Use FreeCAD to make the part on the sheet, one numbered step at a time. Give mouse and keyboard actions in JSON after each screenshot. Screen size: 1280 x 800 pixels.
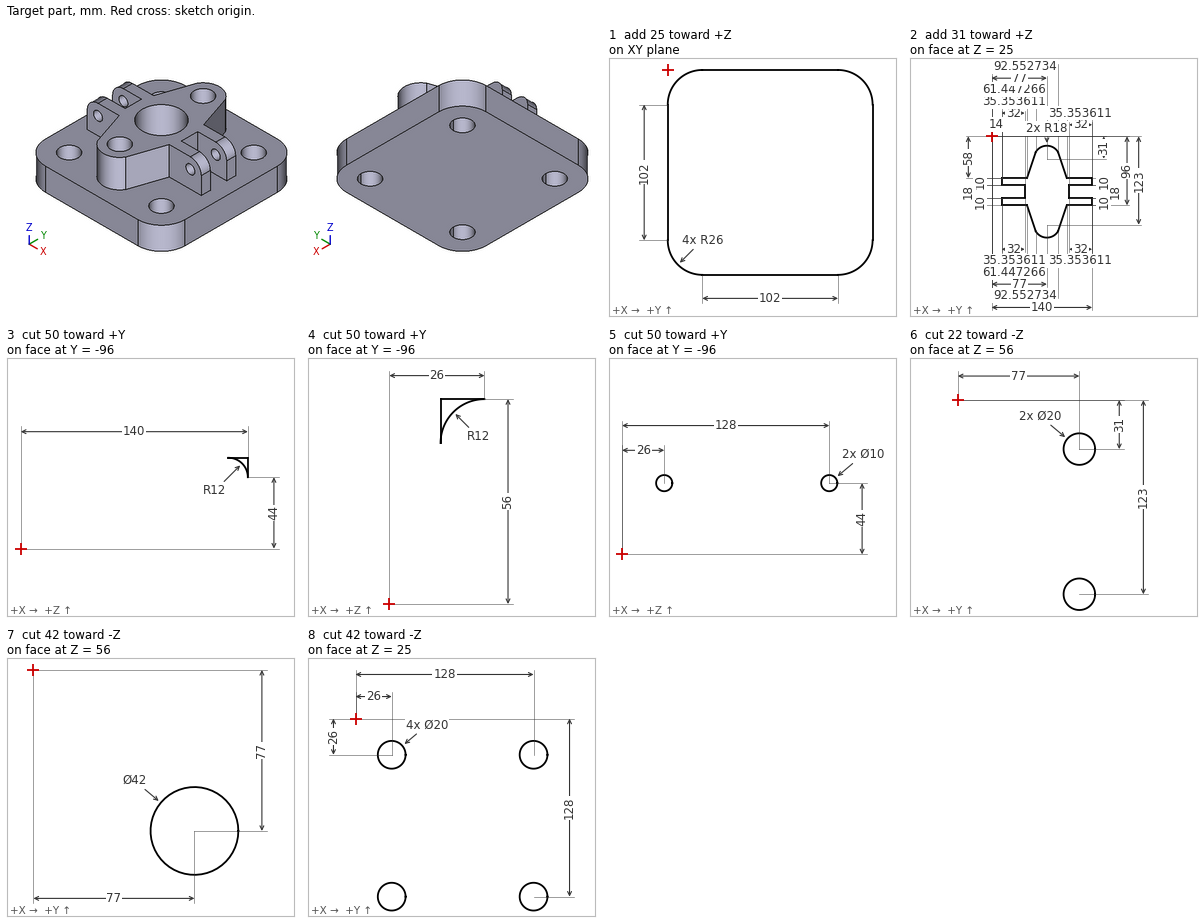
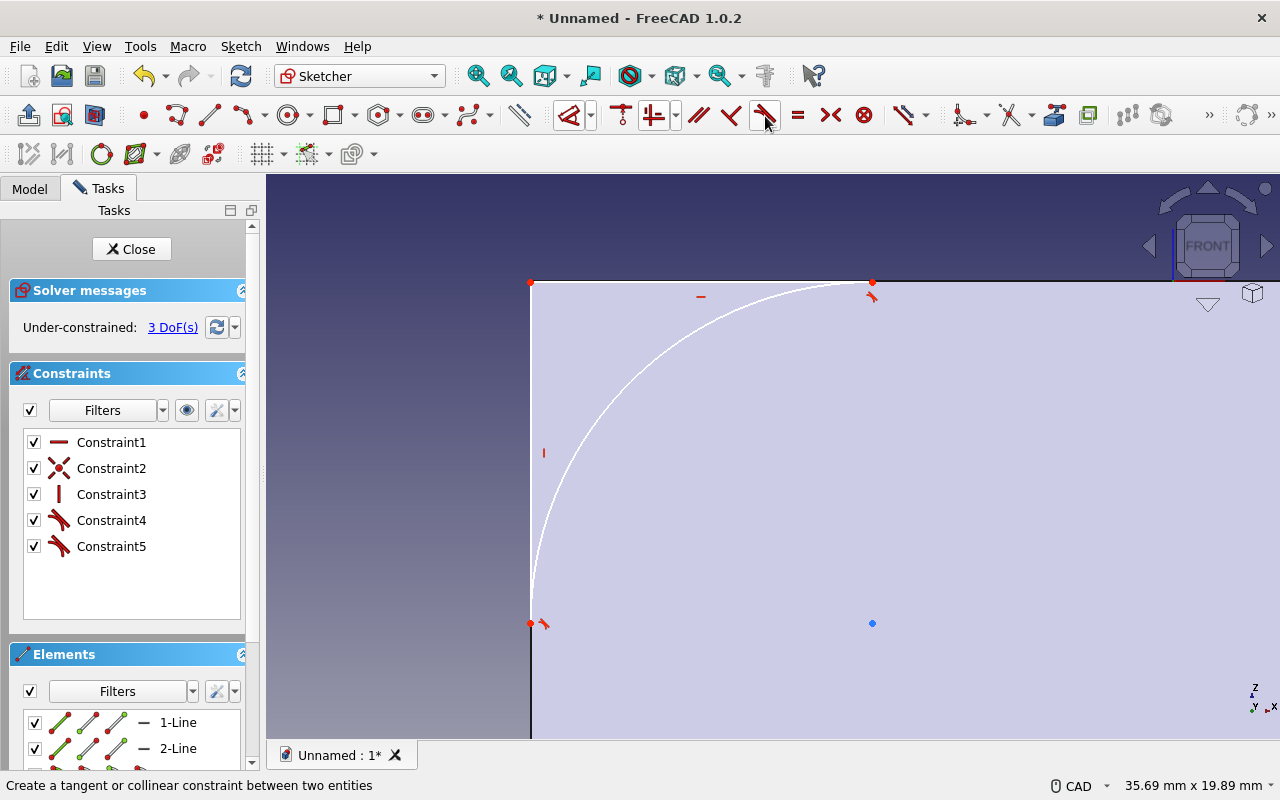
{"action": "left_click", "coordinate": [717, 319]}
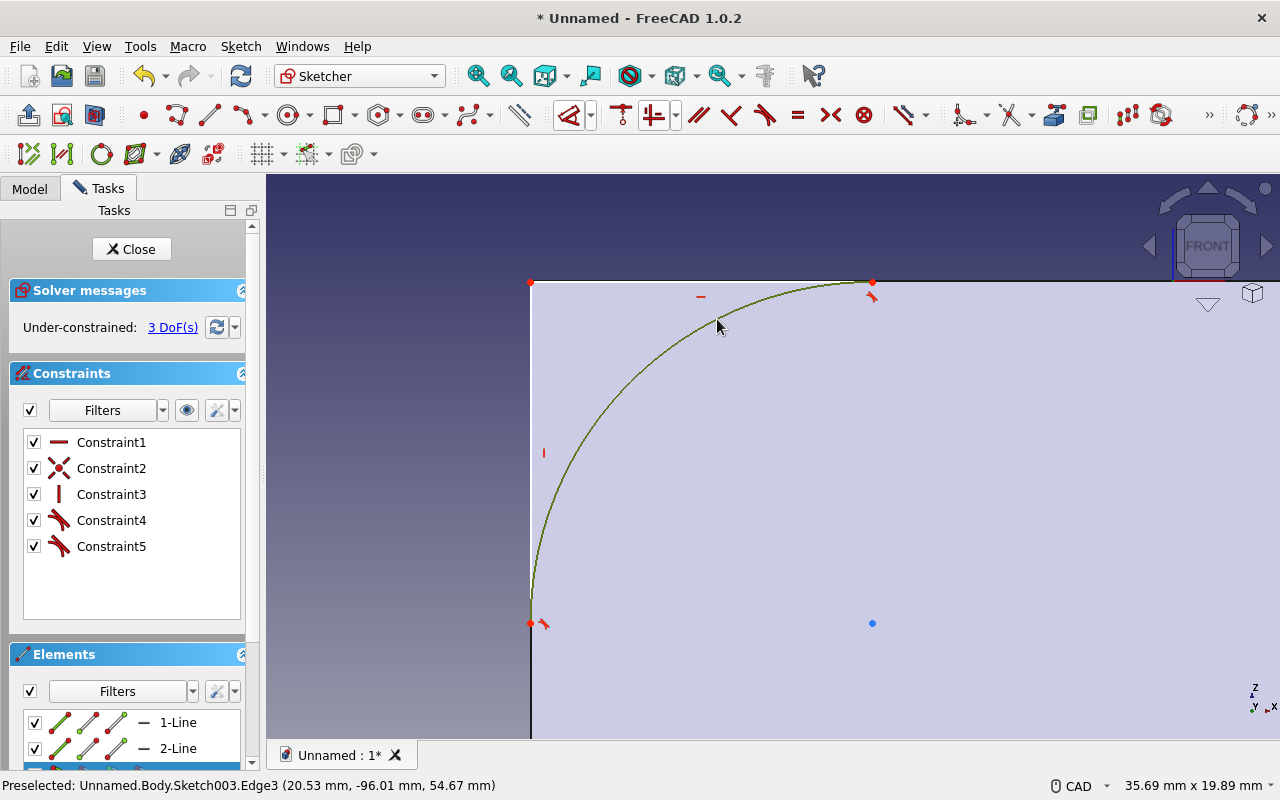
{"action": "key", "text": "k r"}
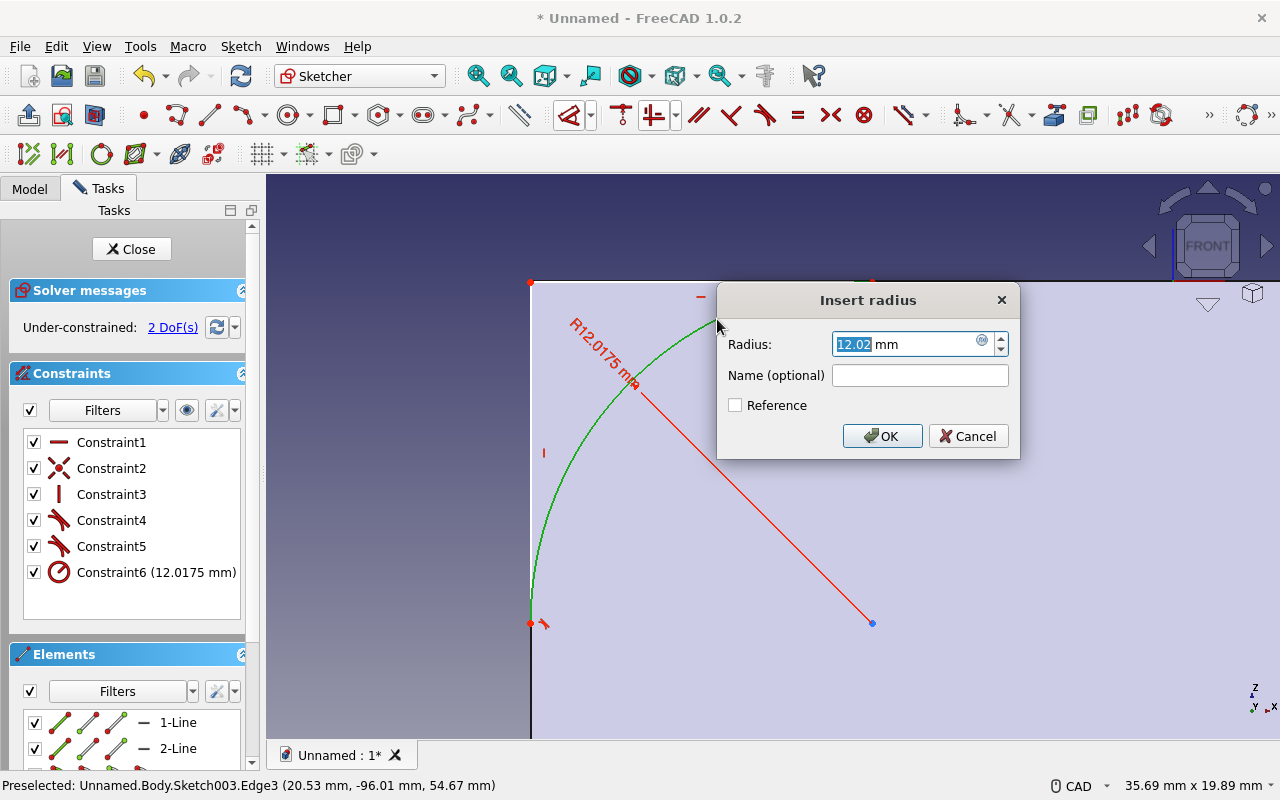
{"action": "type", "text": "12"}
{"action": "key", "text": "Return"}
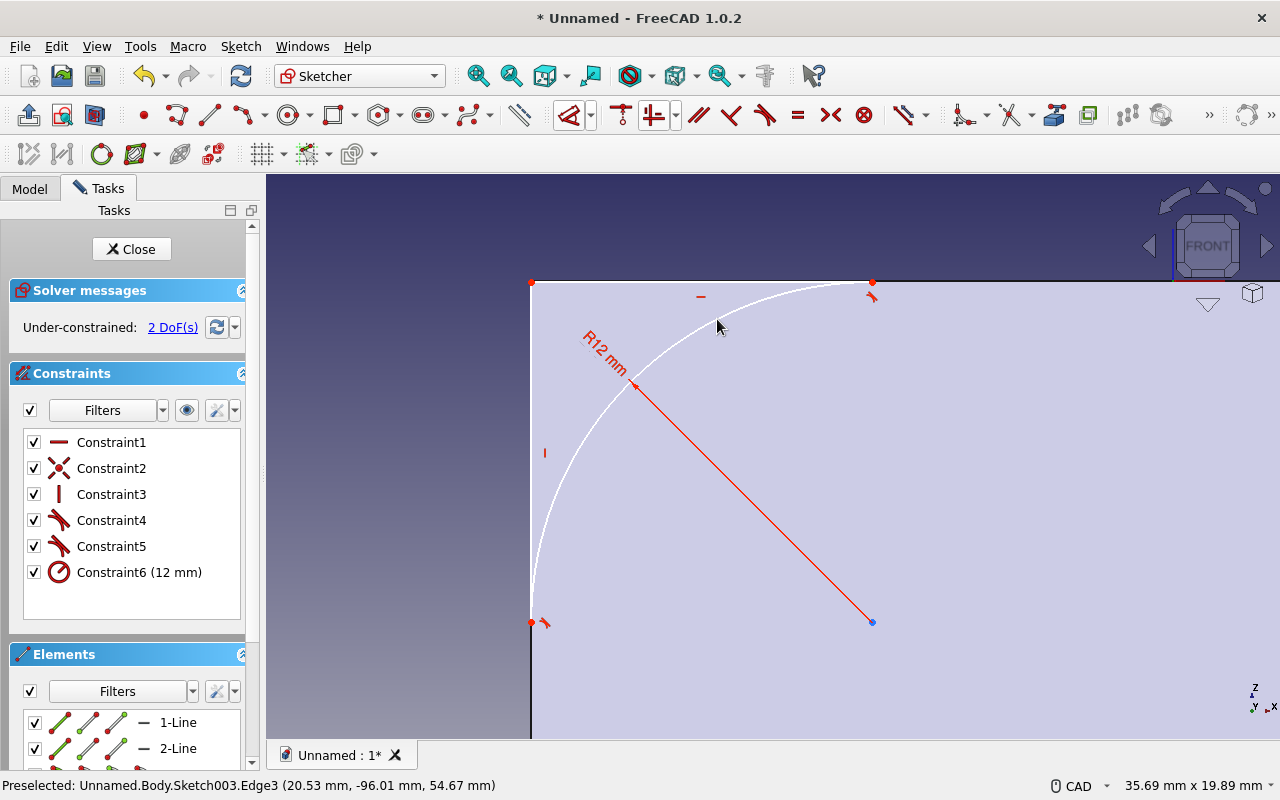
{"action": "left_click", "coordinate": [872, 282]}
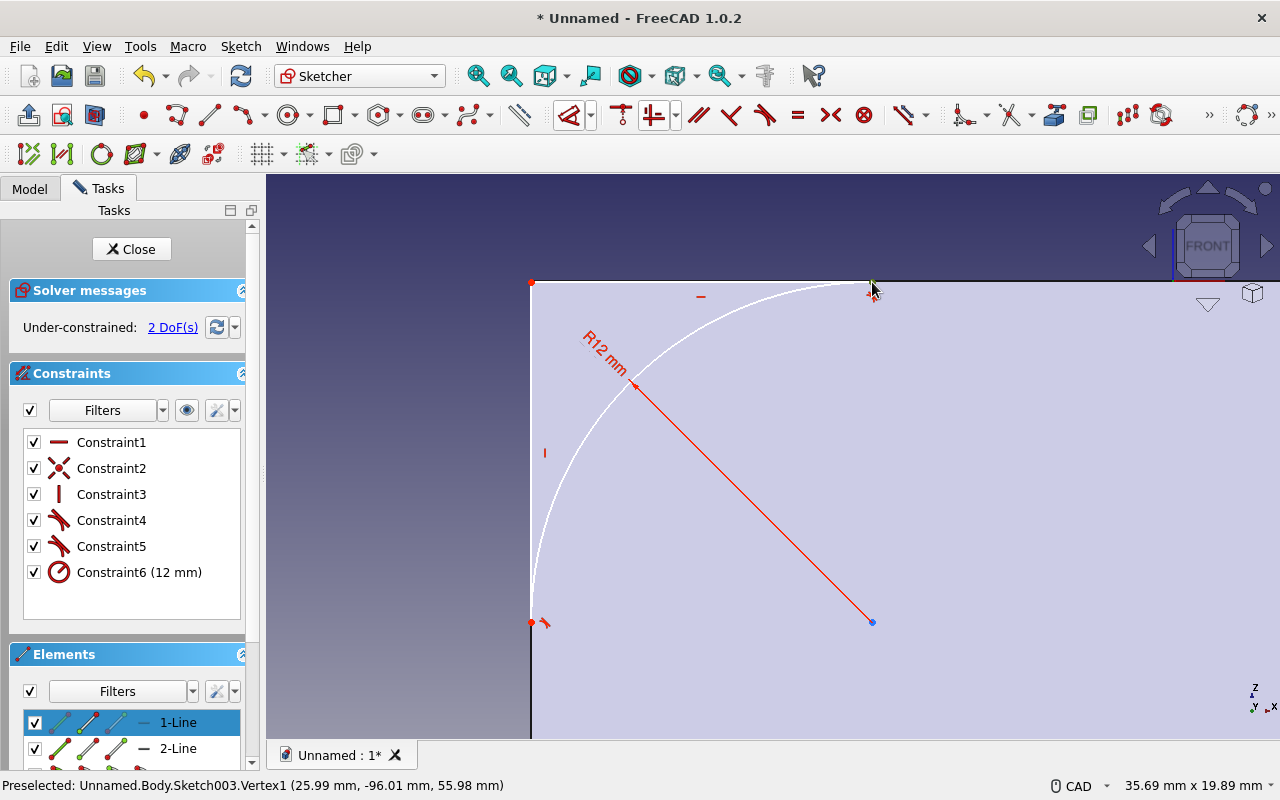
{"action": "key", "text": "l"}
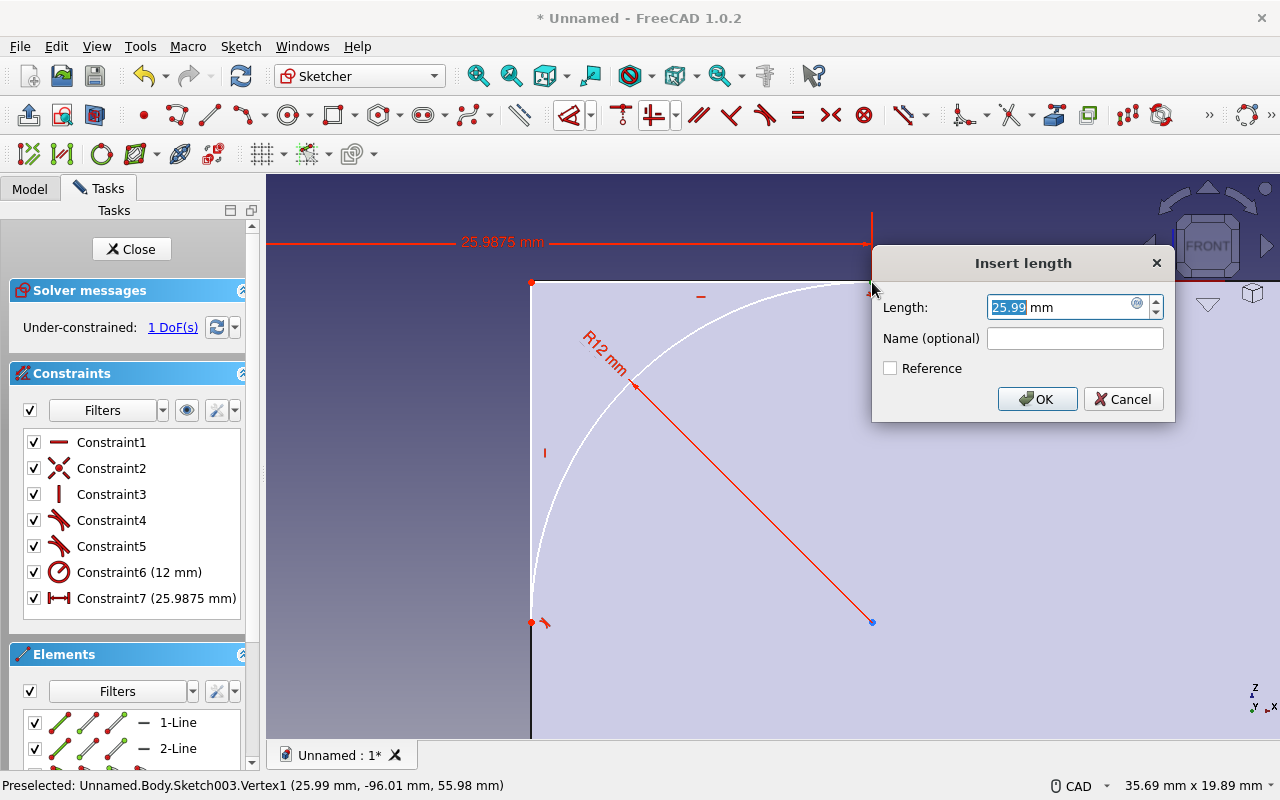
{"action": "type", "text": "26"}
{"action": "key", "text": "Return"}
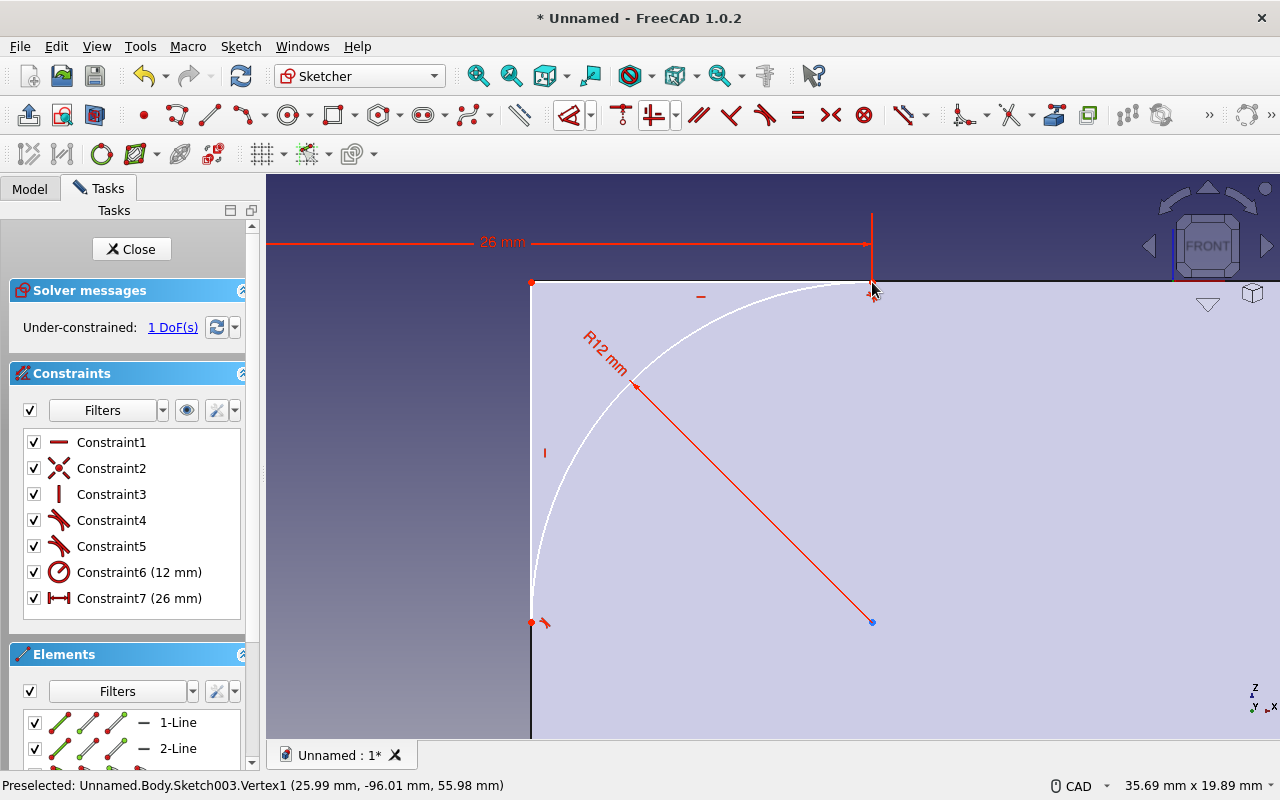
{"action": "left_click", "coordinate": [872, 282]}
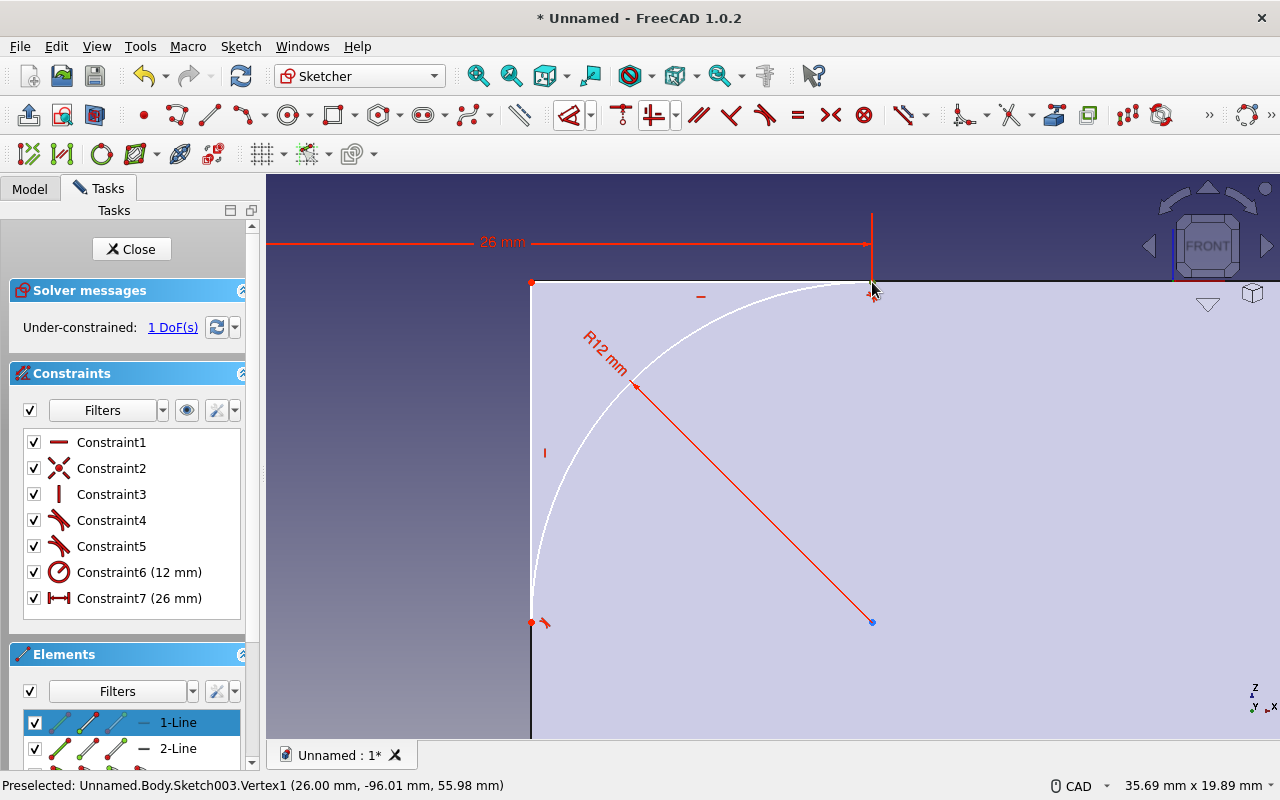
{"action": "left_click", "coordinate": [590, 116]}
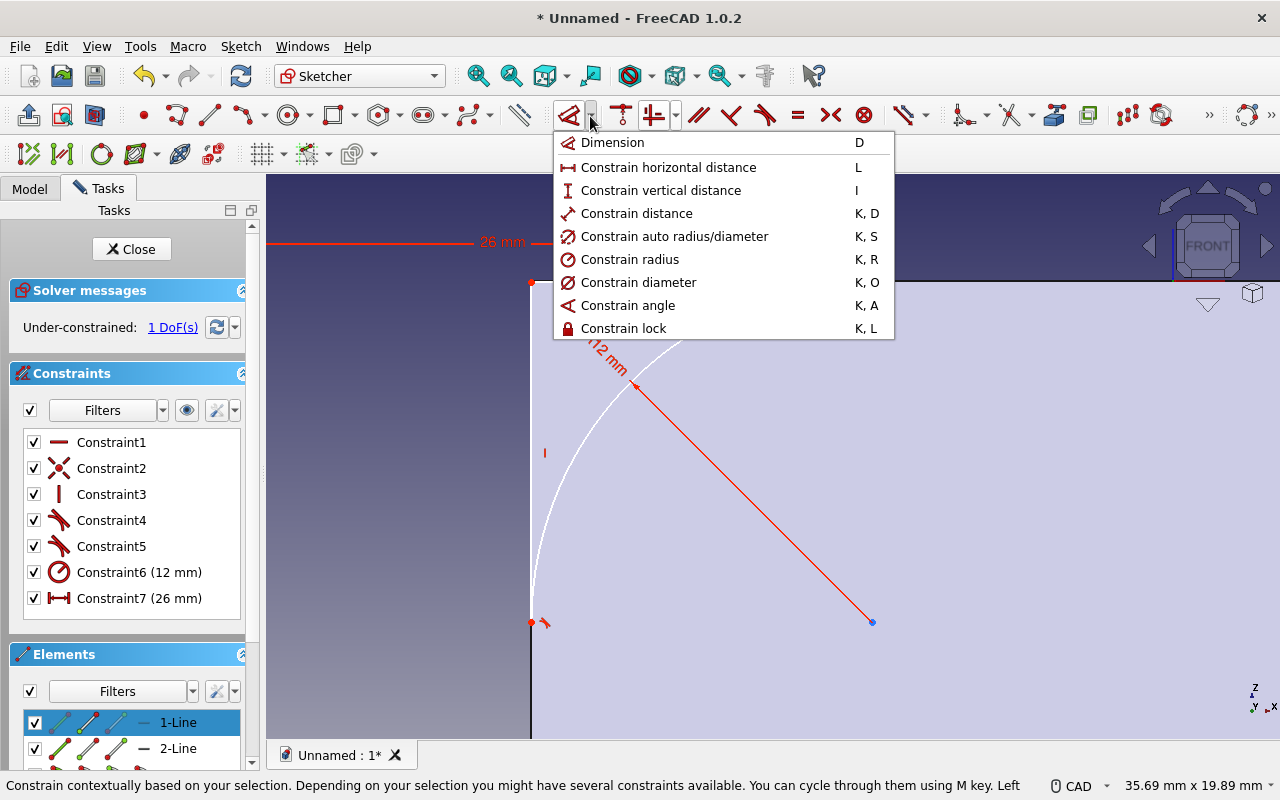
{"action": "left_click", "coordinate": [724, 190]}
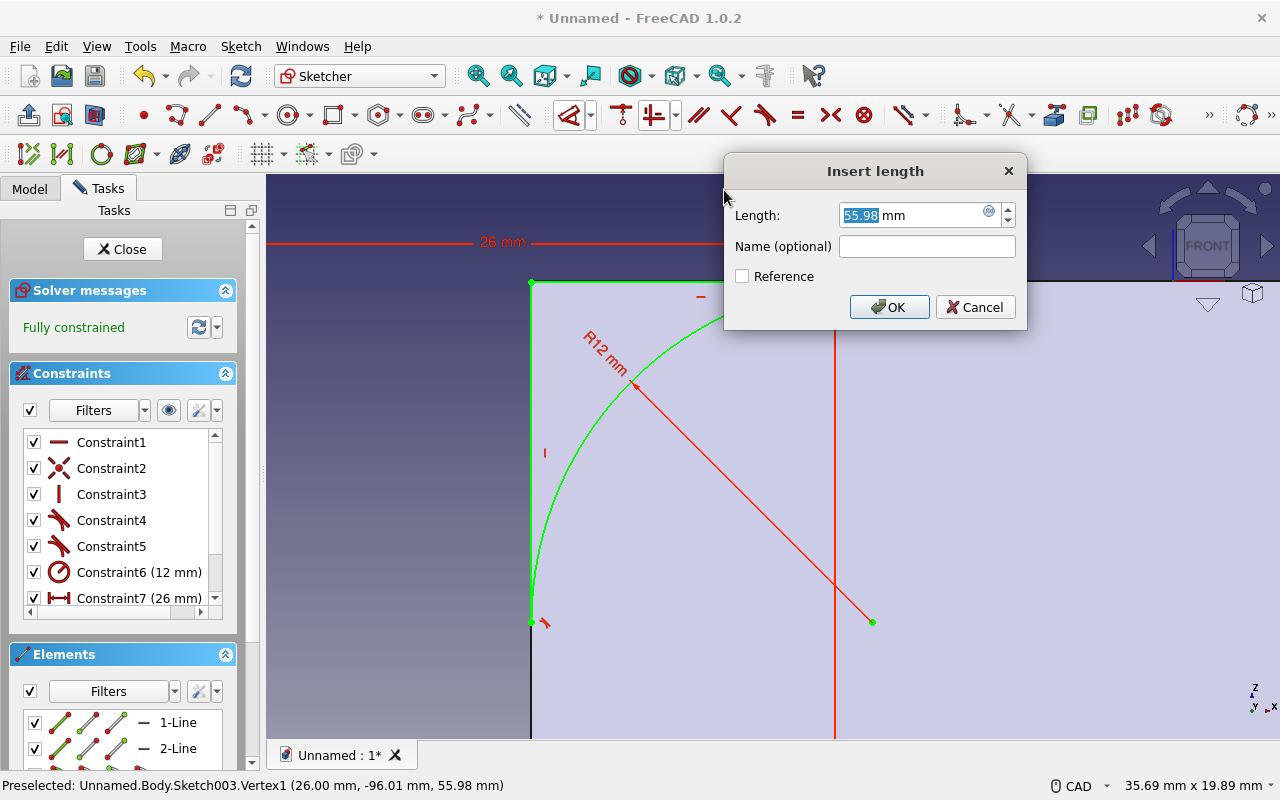
{"action": "type", "text": "56"}
{"action": "key", "text": "Return"}